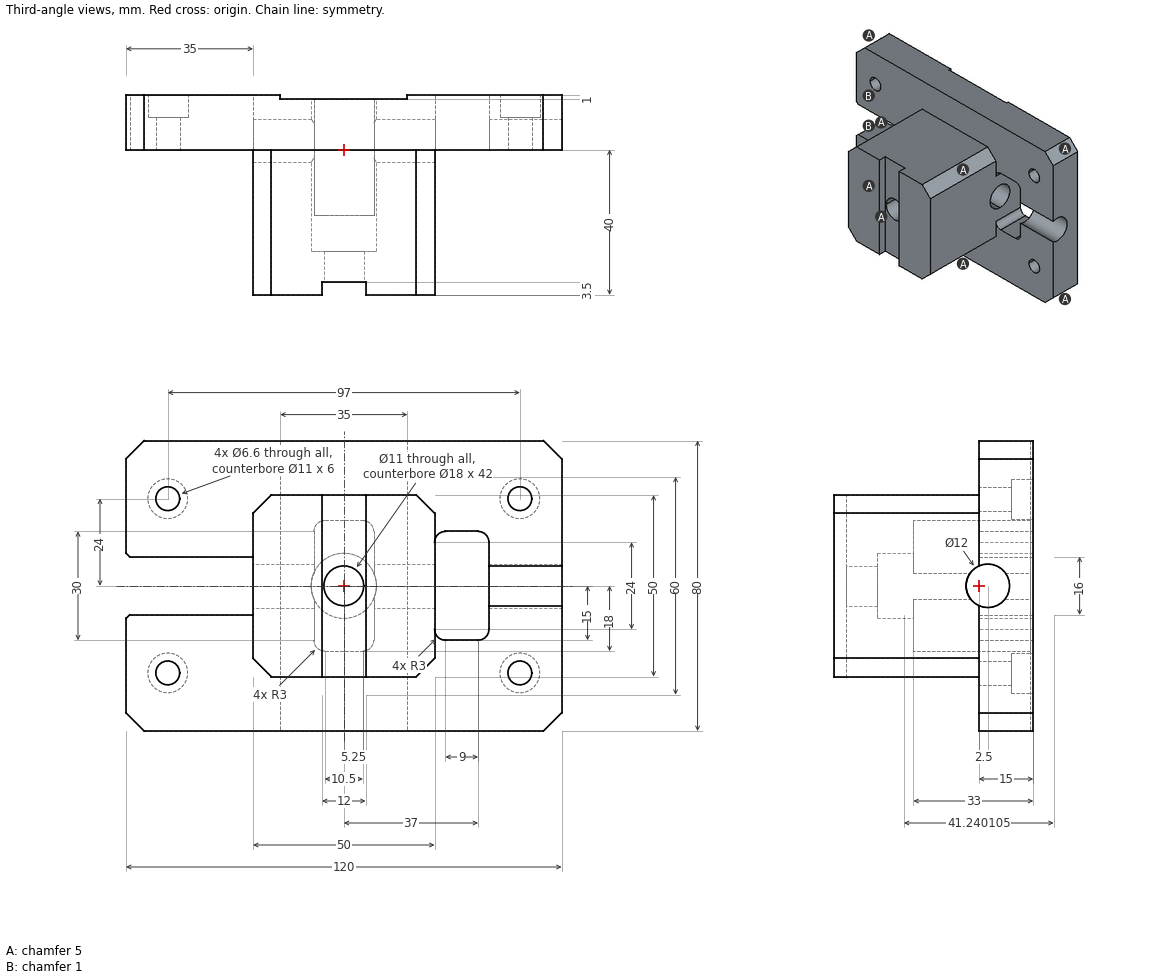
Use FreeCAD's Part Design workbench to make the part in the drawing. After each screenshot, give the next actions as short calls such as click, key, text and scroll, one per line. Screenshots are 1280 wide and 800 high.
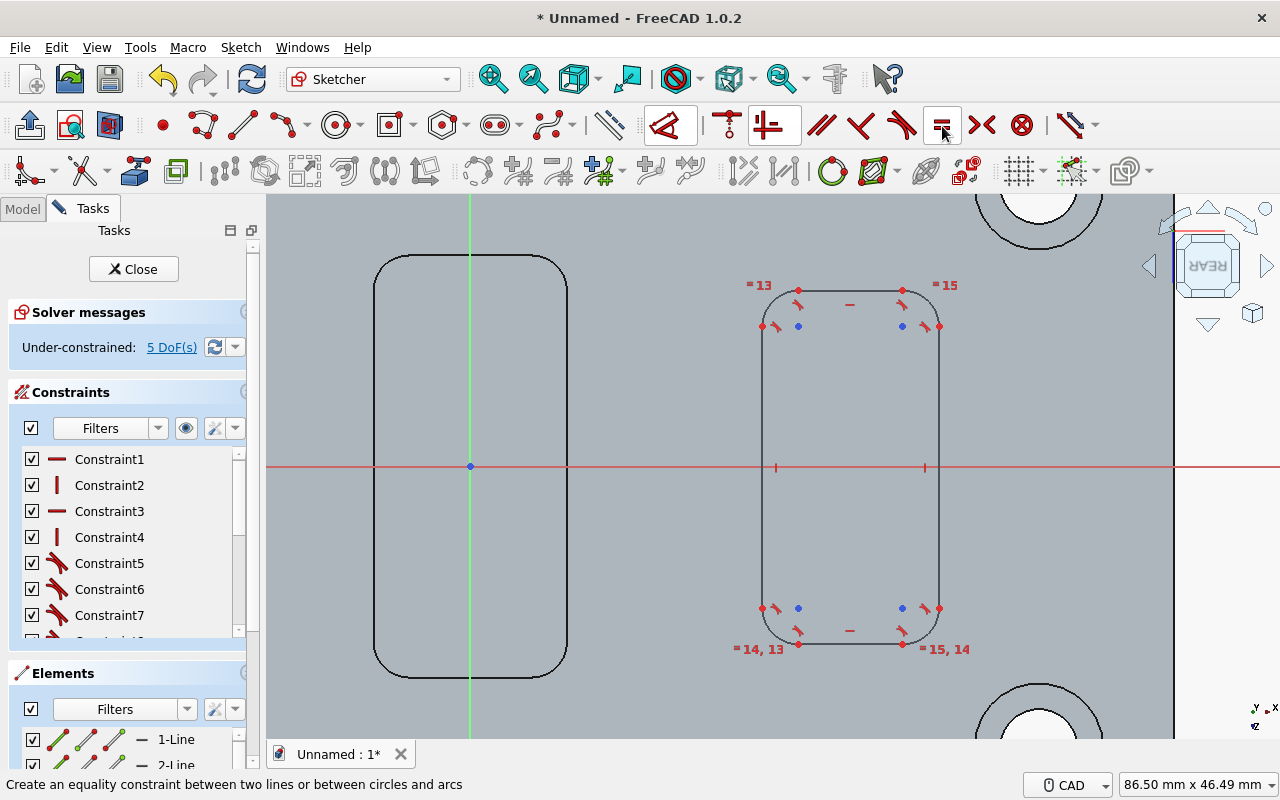
click(782, 295)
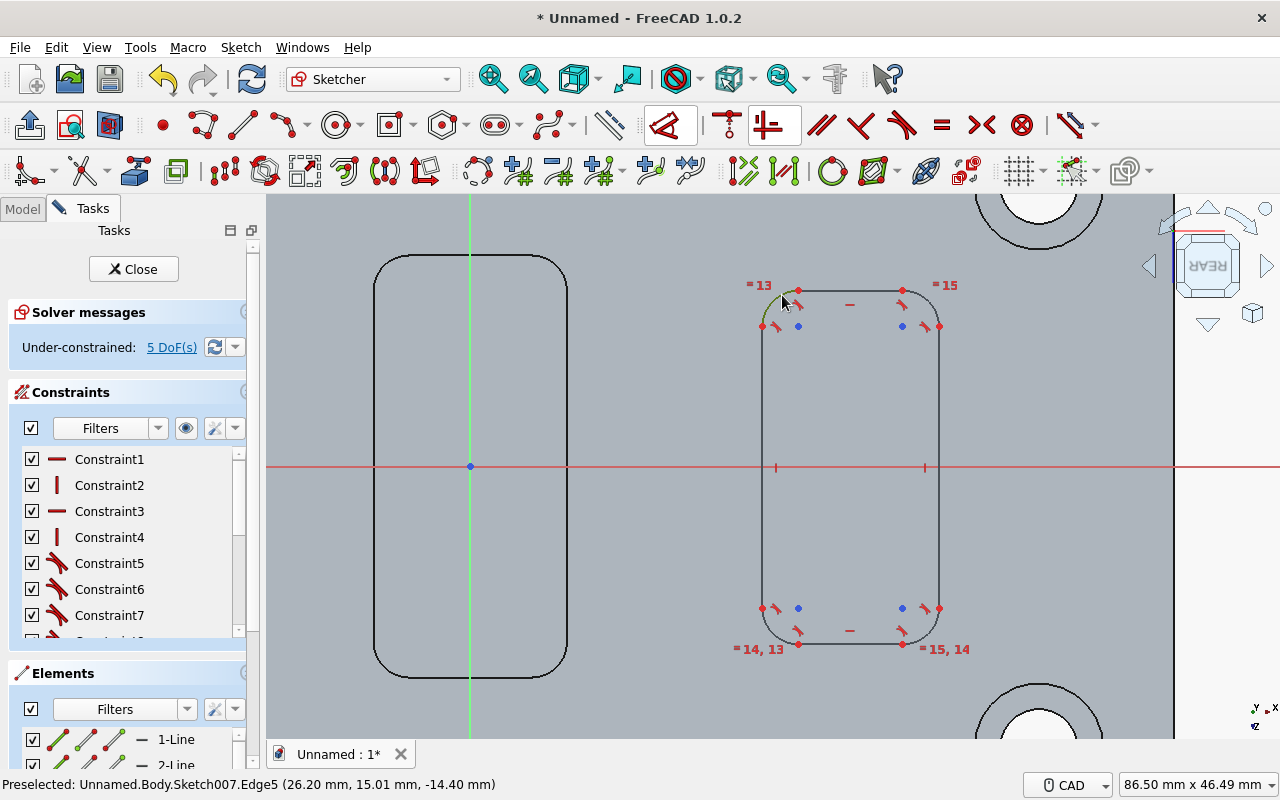
key(k)
key(r)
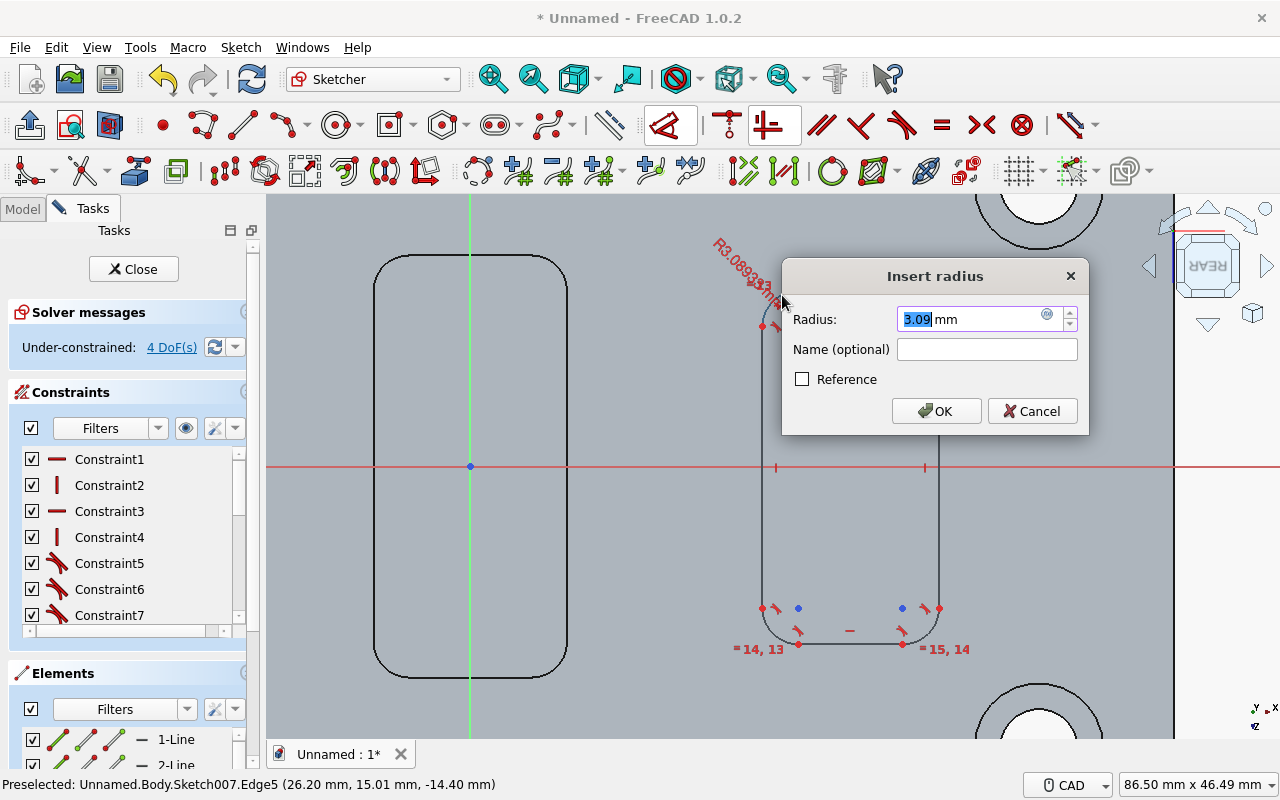
text(3)
key(Return)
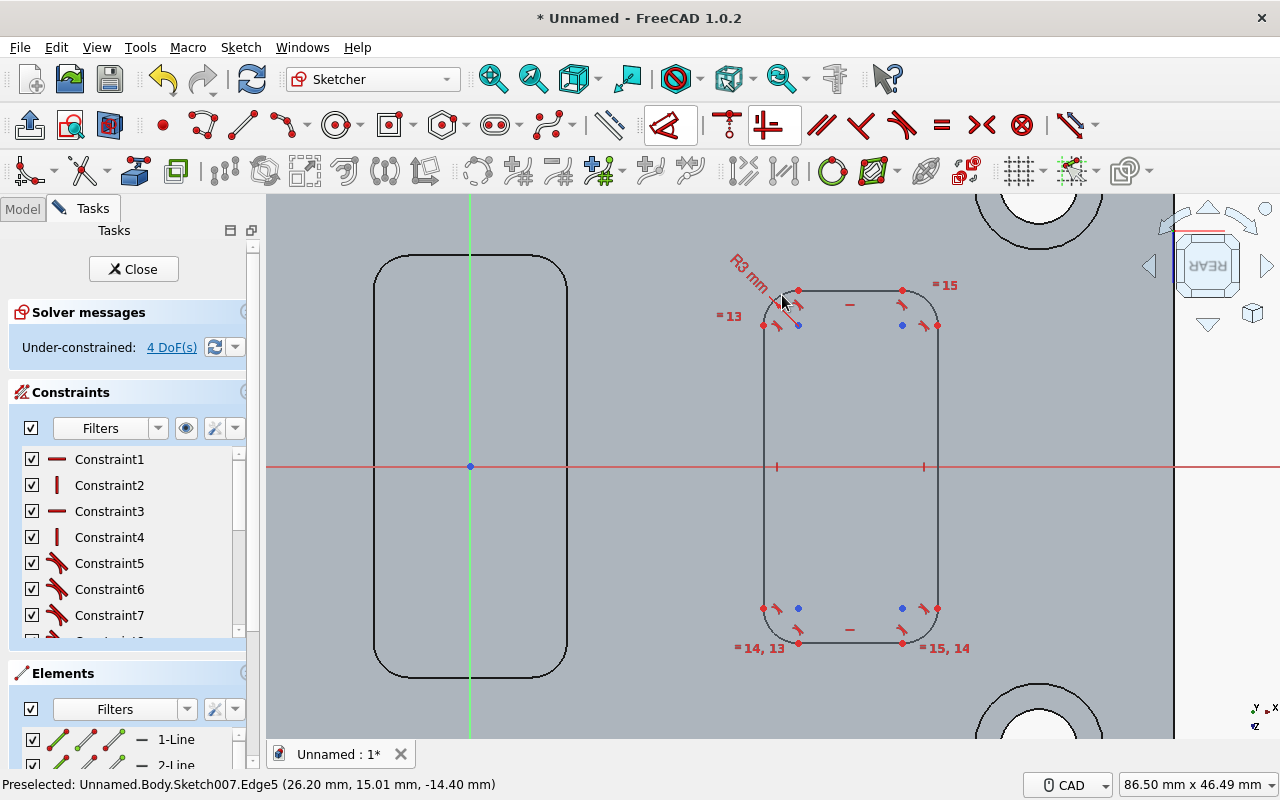
click(872, 291)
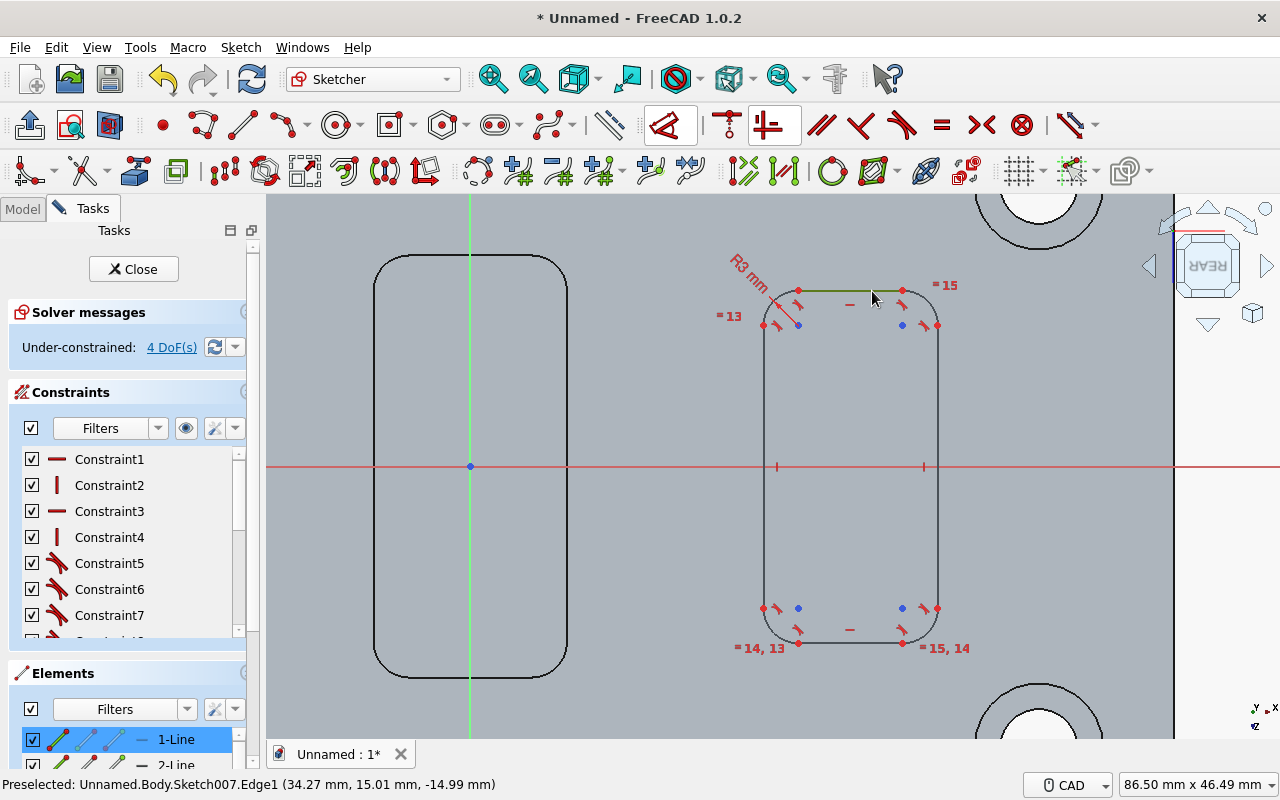
click(692, 126)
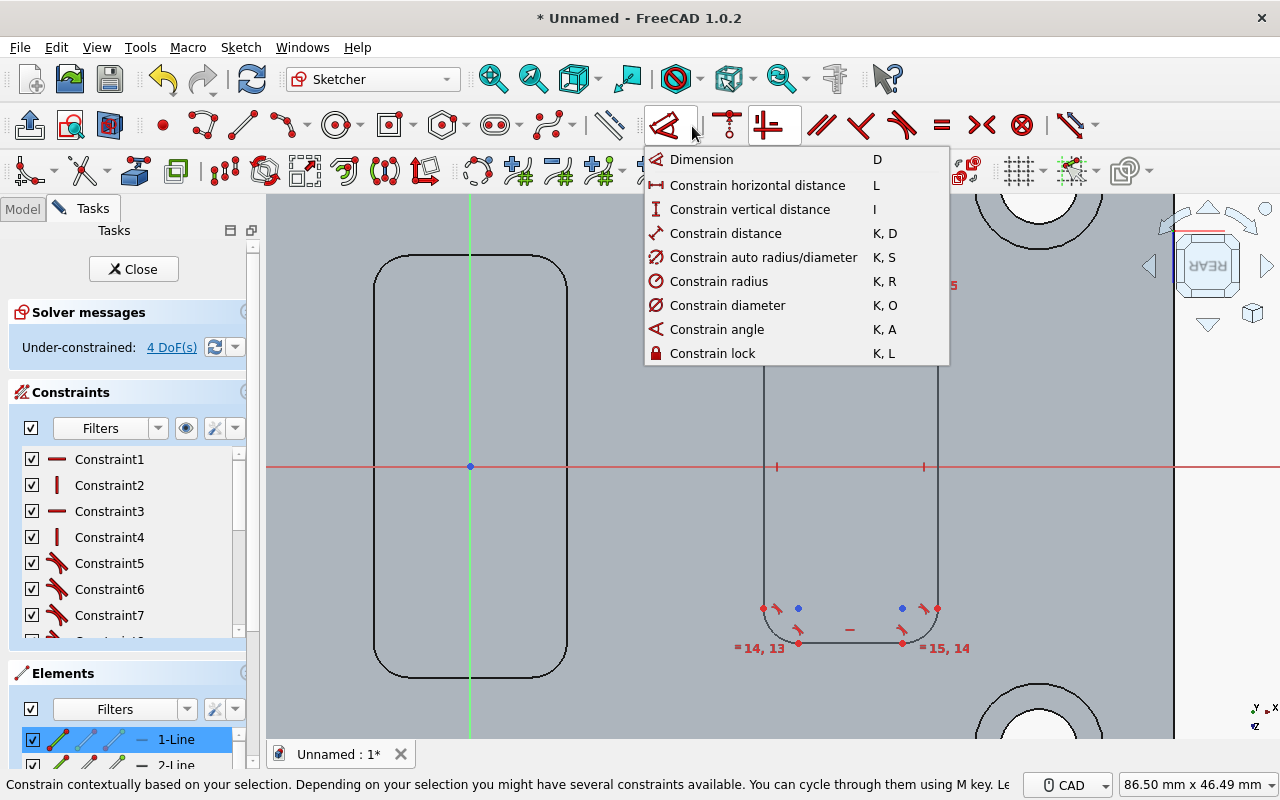
click(797, 185)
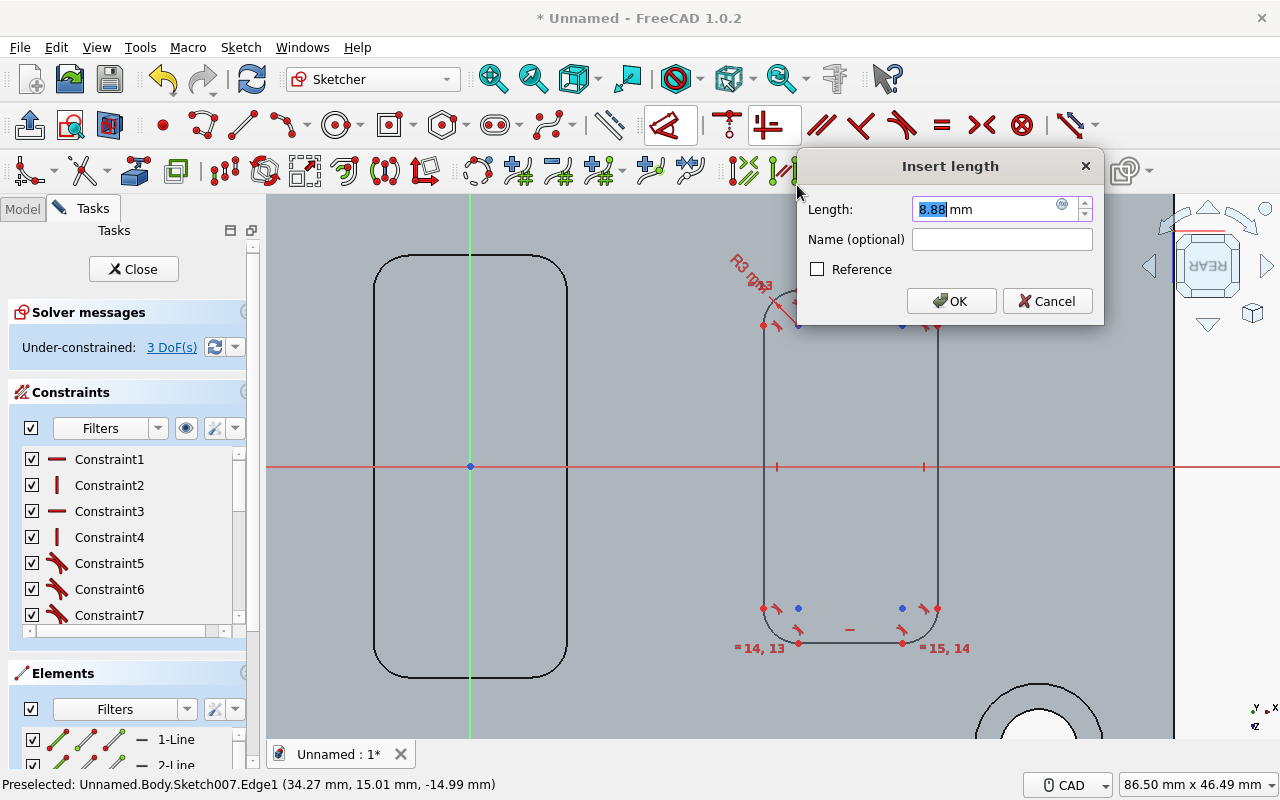
text(9)
key(Return)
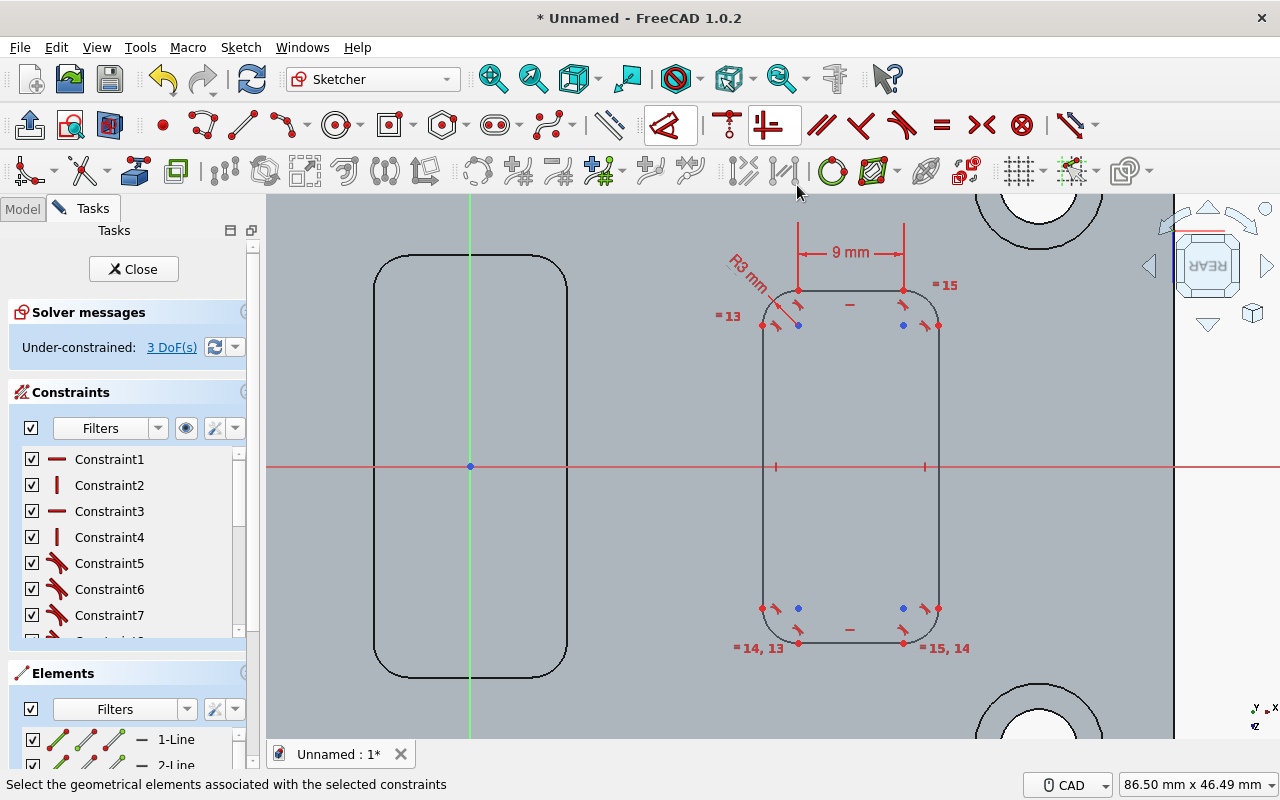
click(763, 411)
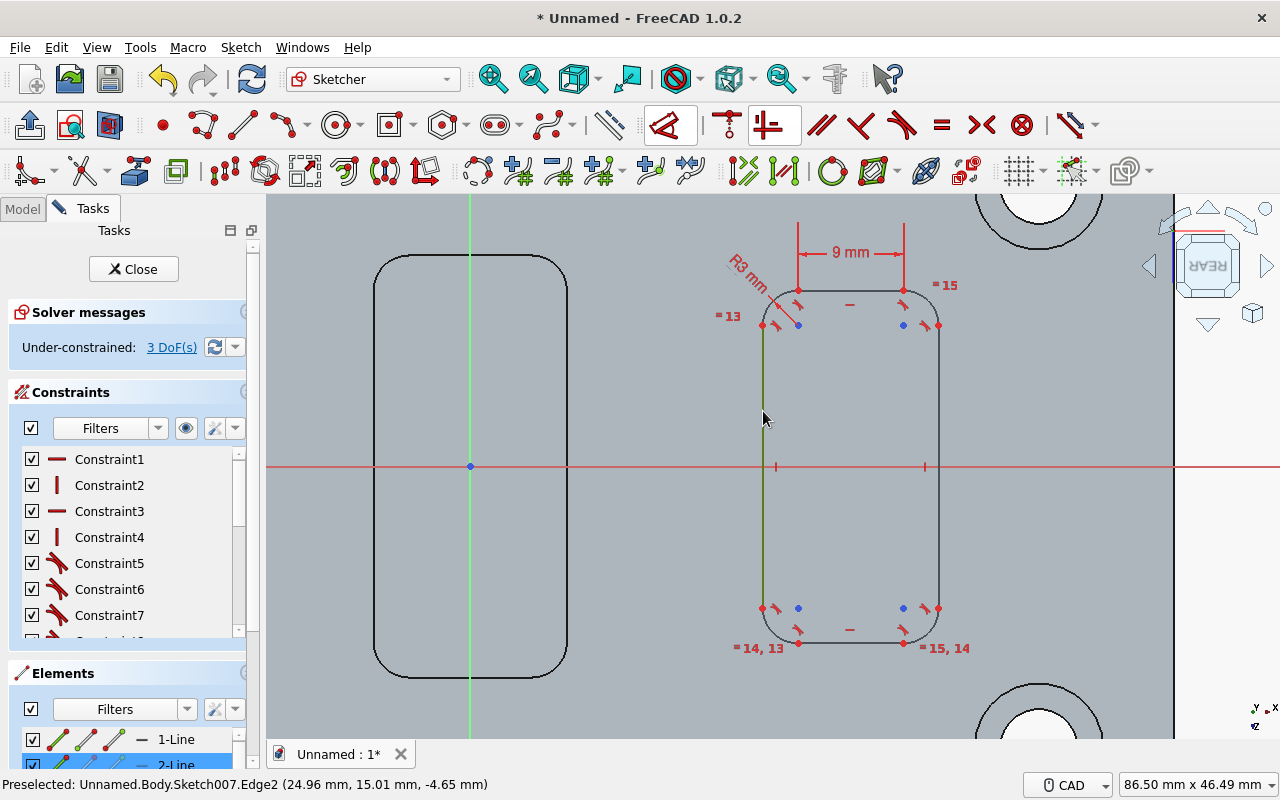
click(692, 126)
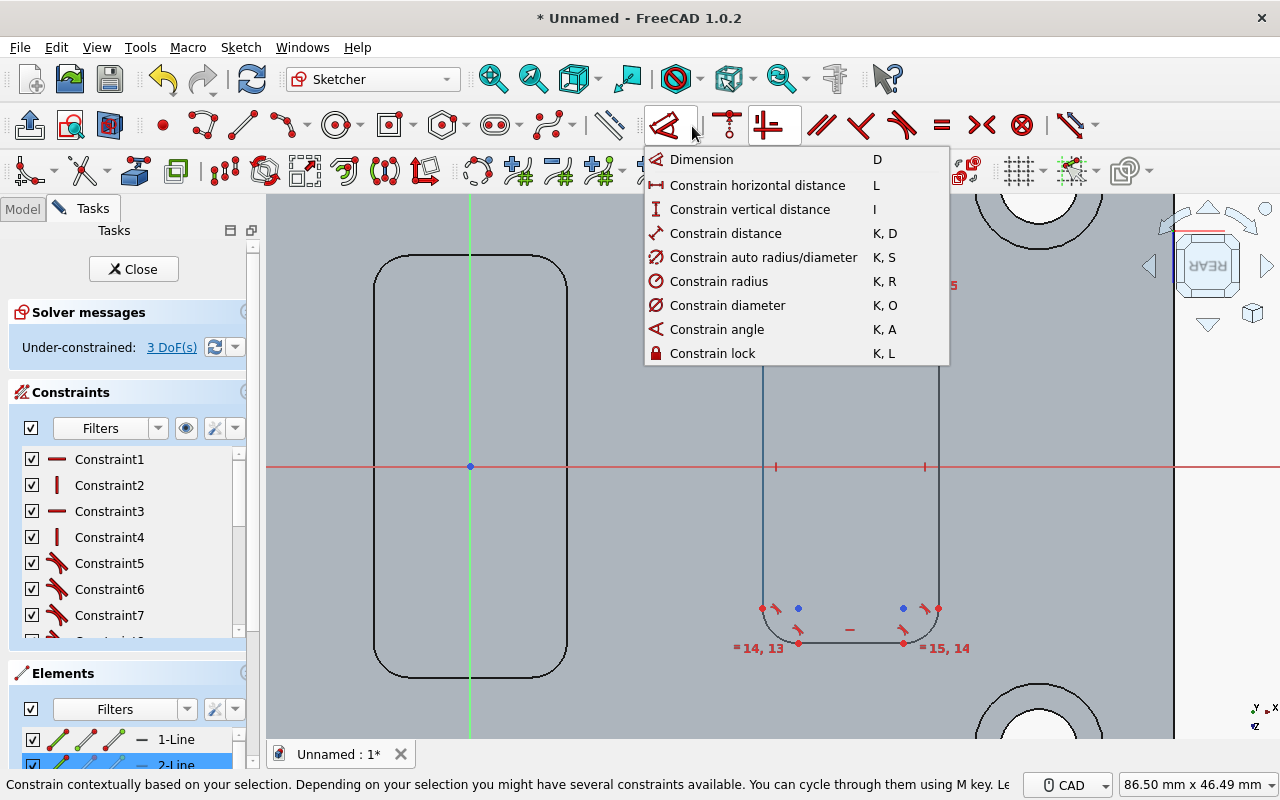
click(797, 209)